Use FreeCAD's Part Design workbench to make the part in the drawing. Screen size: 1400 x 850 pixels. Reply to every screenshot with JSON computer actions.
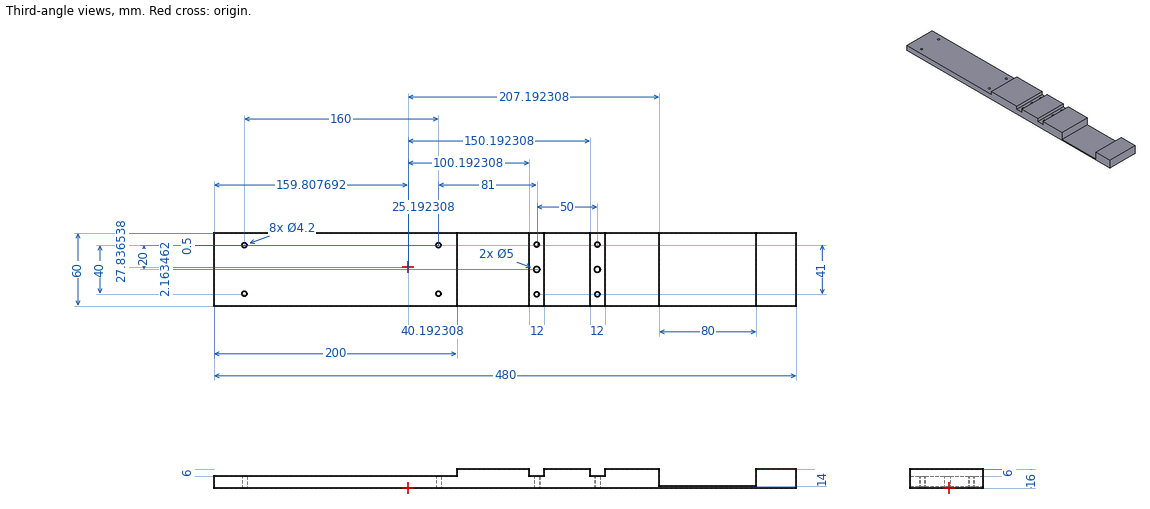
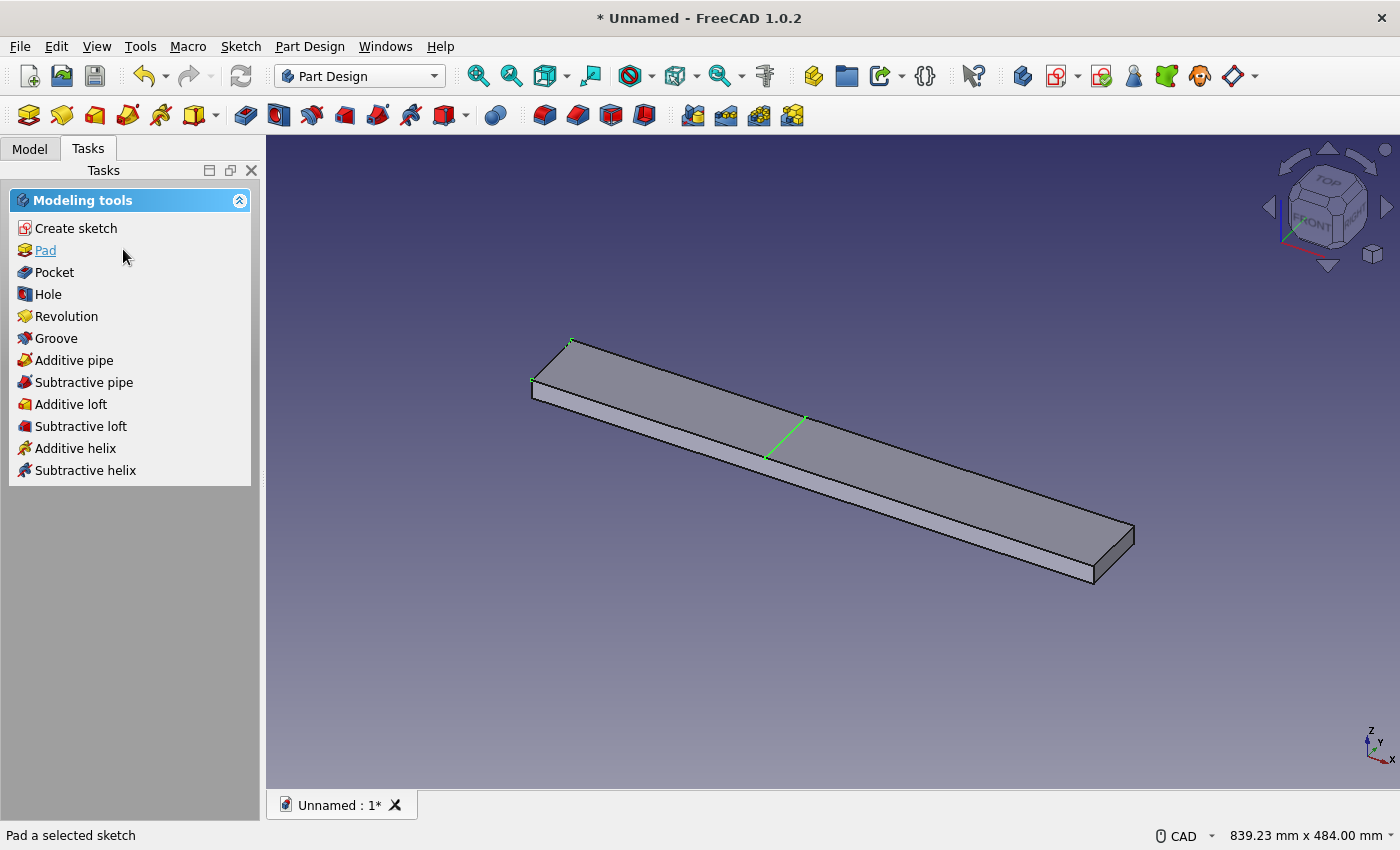
{"action": "left_click", "coordinate": [246, 116]}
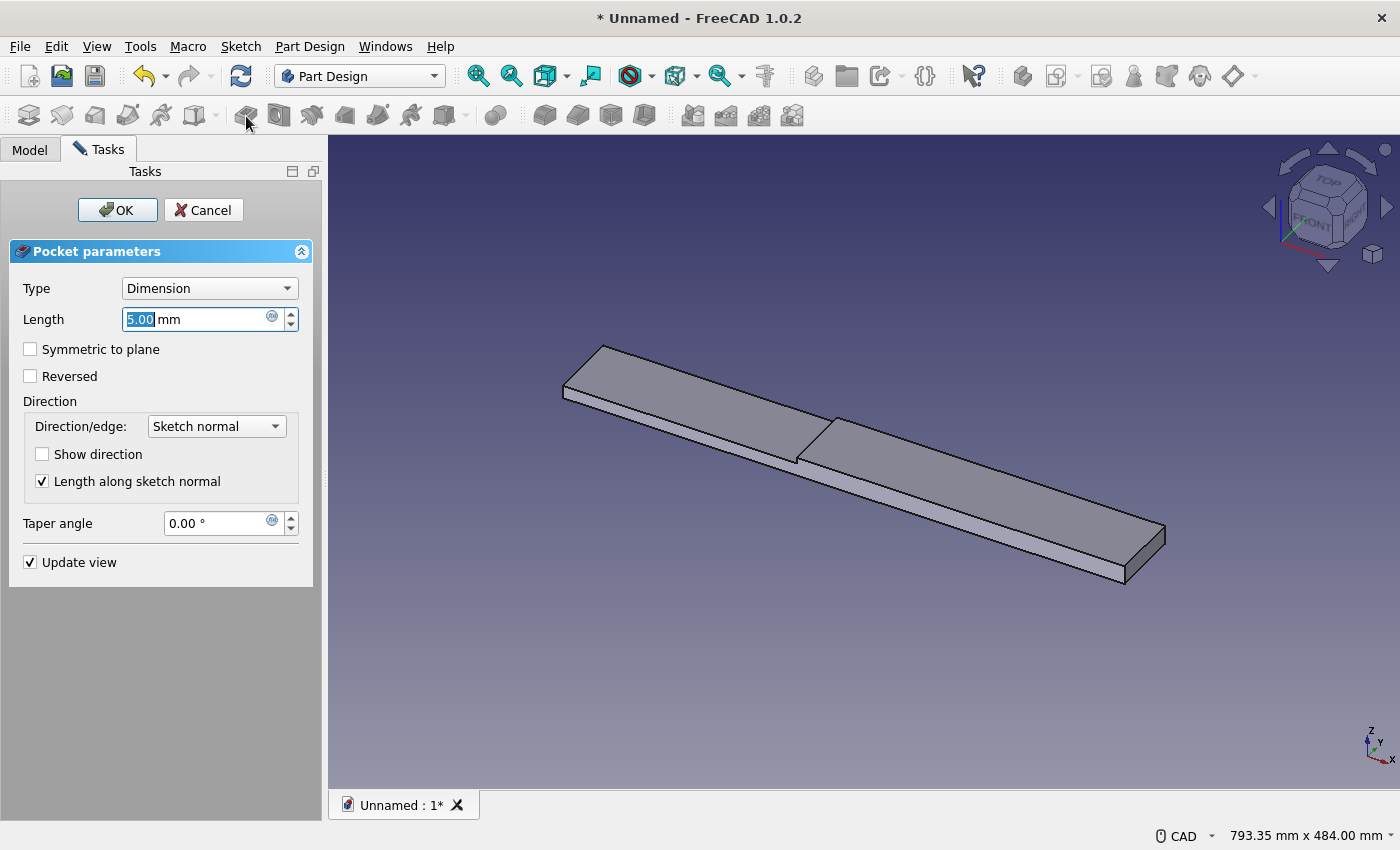
{"action": "type", "text": "6"}
{"action": "key", "text": "Tab"}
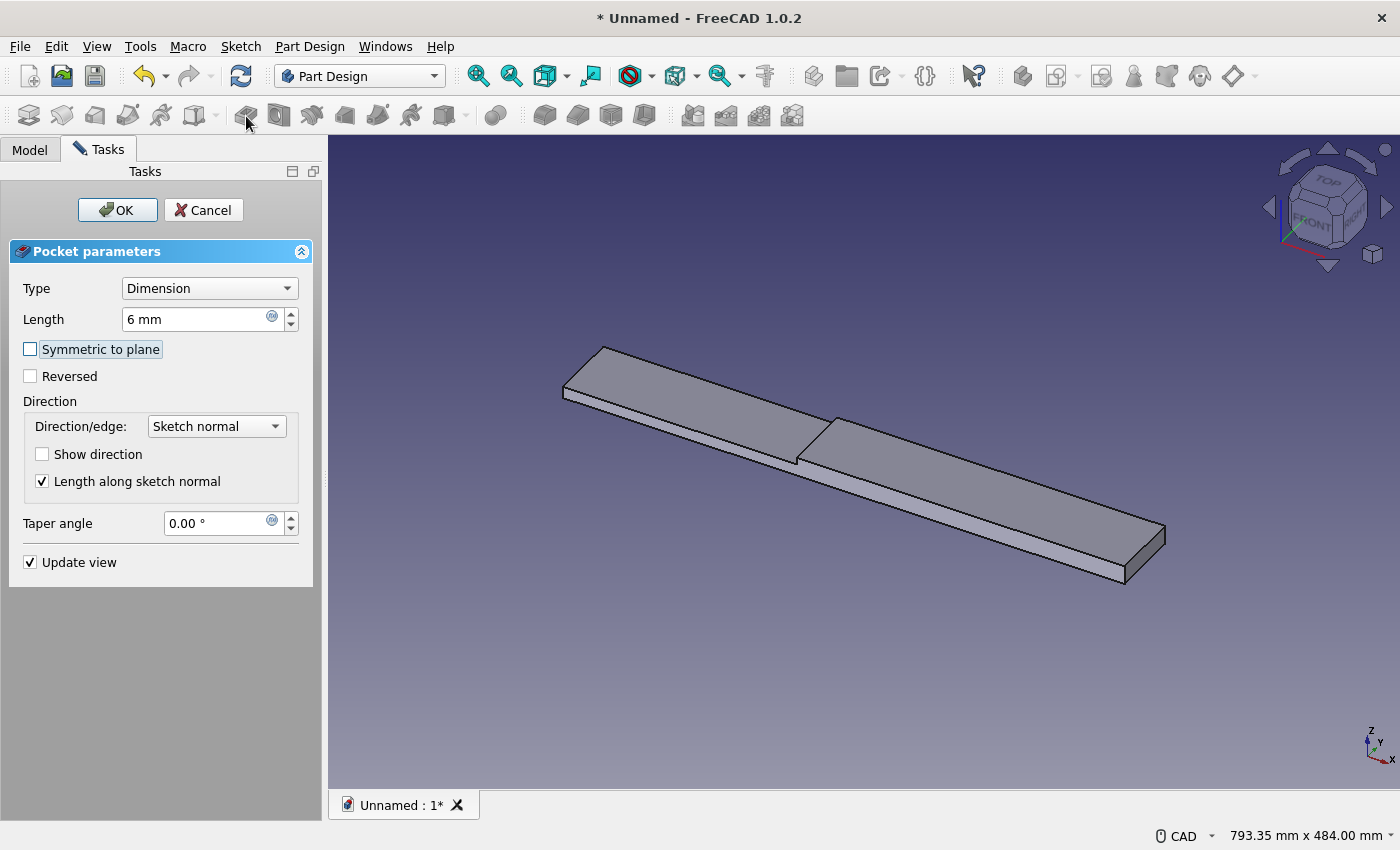
{"action": "left_click", "coordinate": [118, 210]}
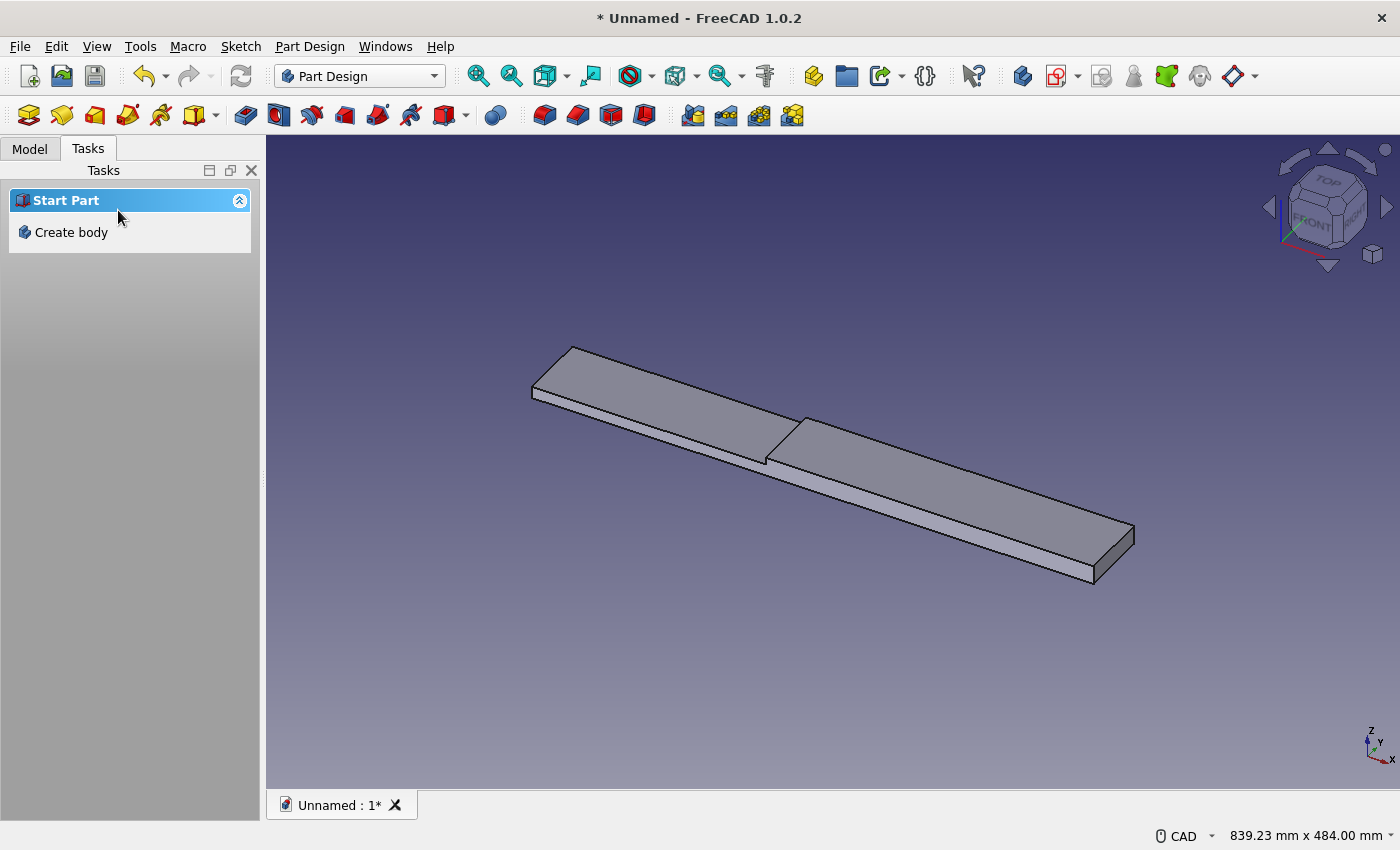
{"action": "left_click", "coordinate": [1044, 522]}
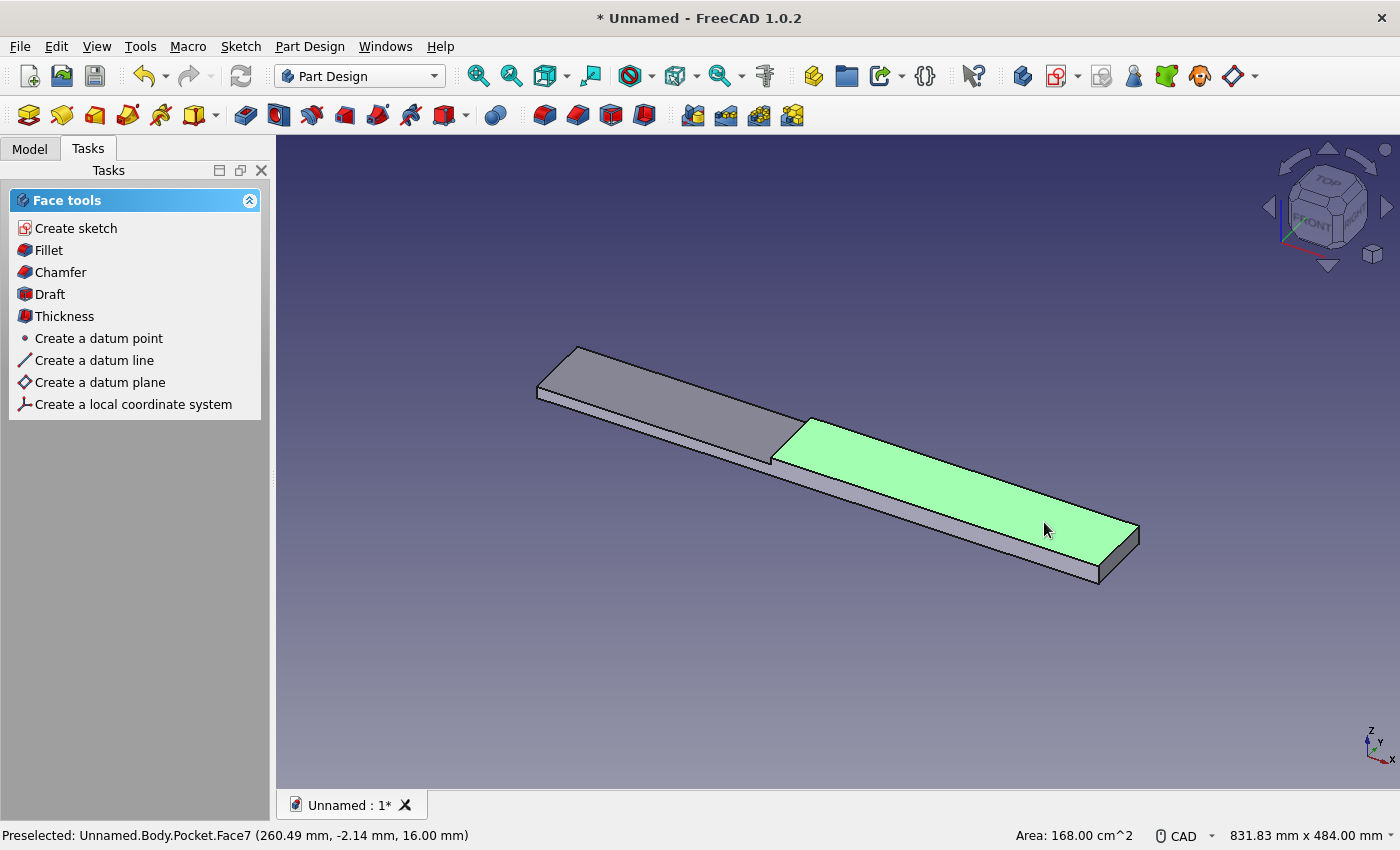
{"action": "left_click", "coordinate": [1056, 76]}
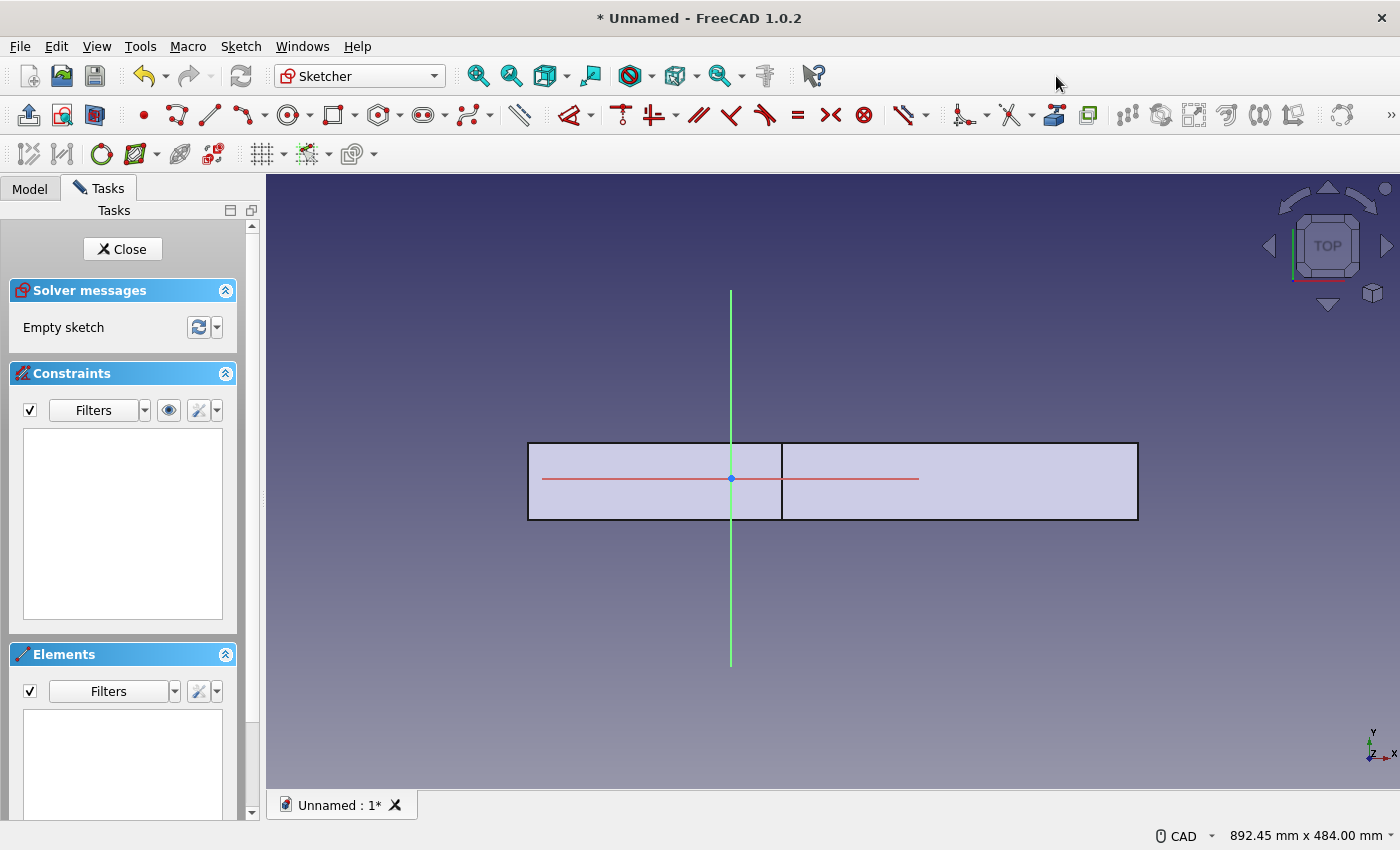
{"action": "scroll", "coordinate": [932, 482], "scroll_direction": "up", "scroll_amount": 8}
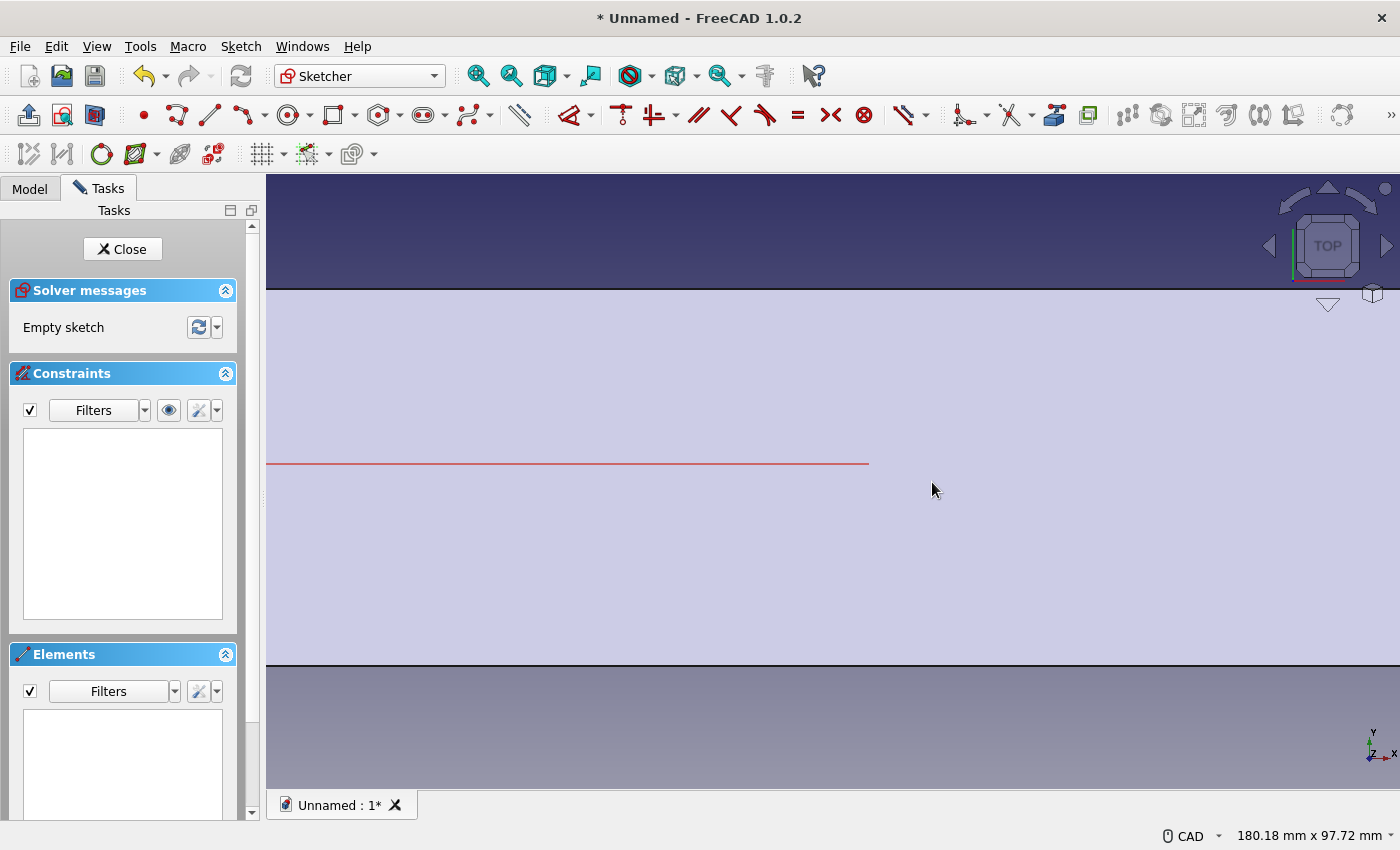
{"action": "left_click", "coordinate": [332, 116]}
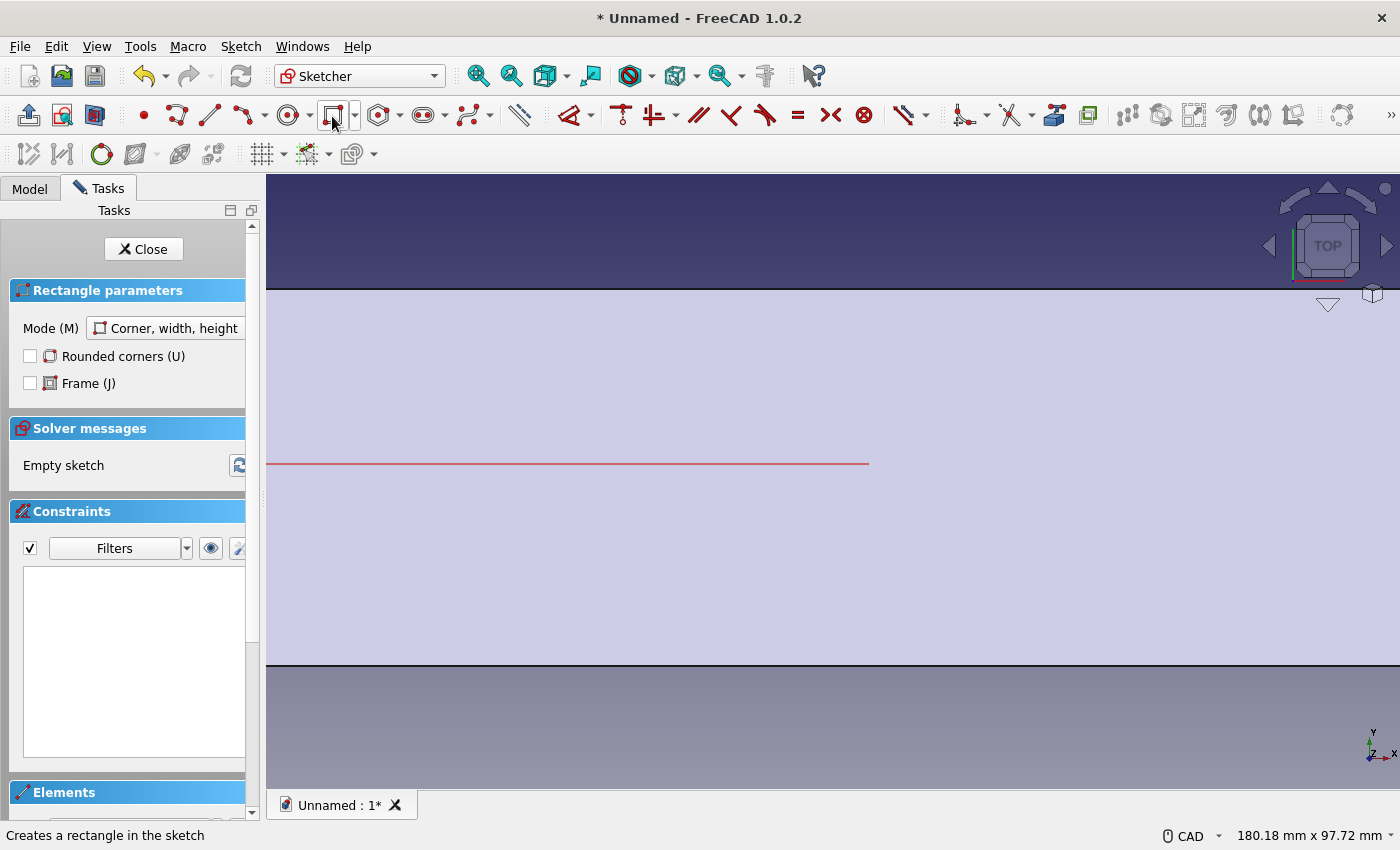
{"action": "left_click", "coordinate": [565, 289]}
{"action": "left_click", "coordinate": [641, 666]}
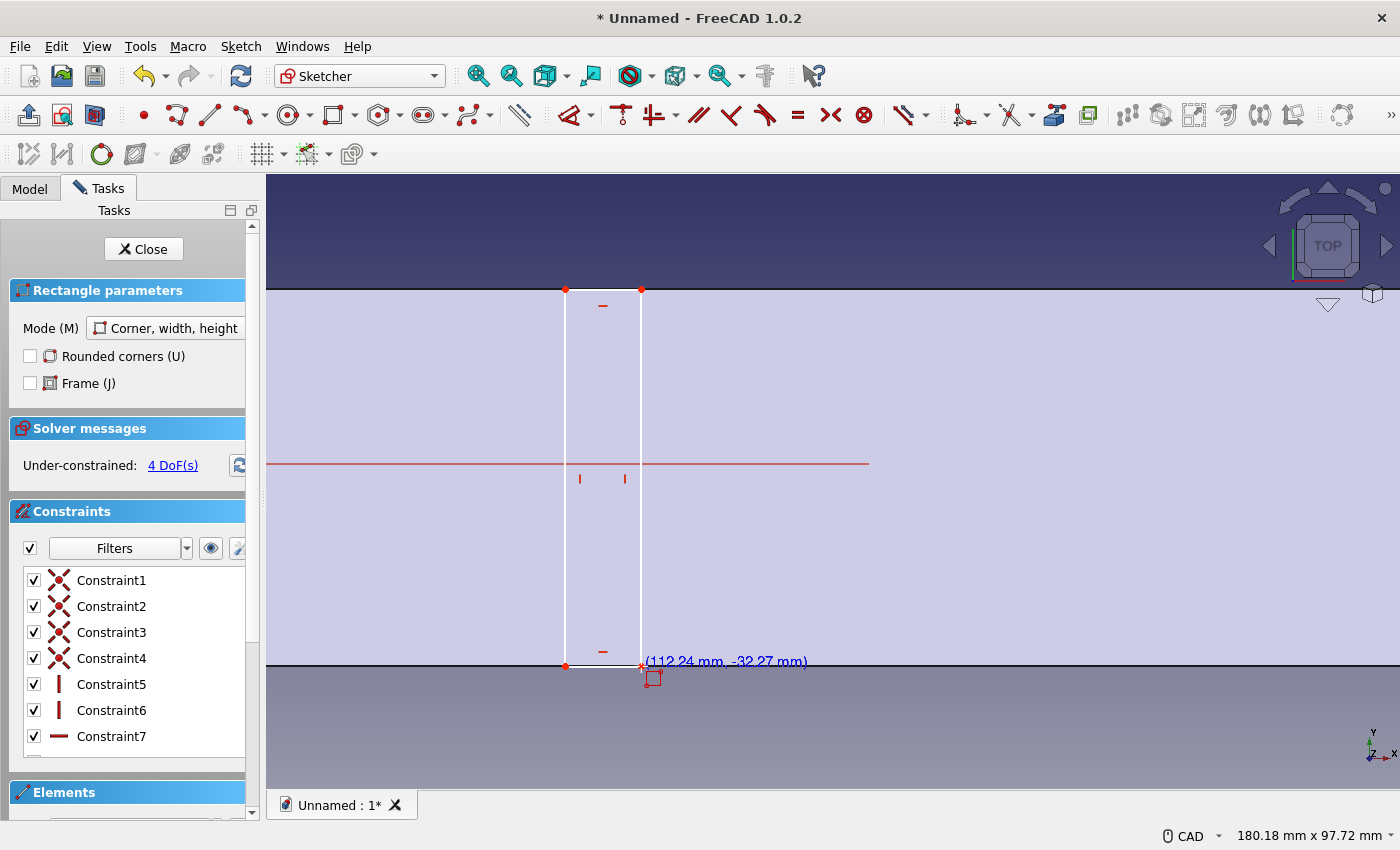
{"action": "left_click", "coordinate": [880, 289]}
{"action": "left_click", "coordinate": [955, 666]}
{"action": "key", "text": "Escape"}